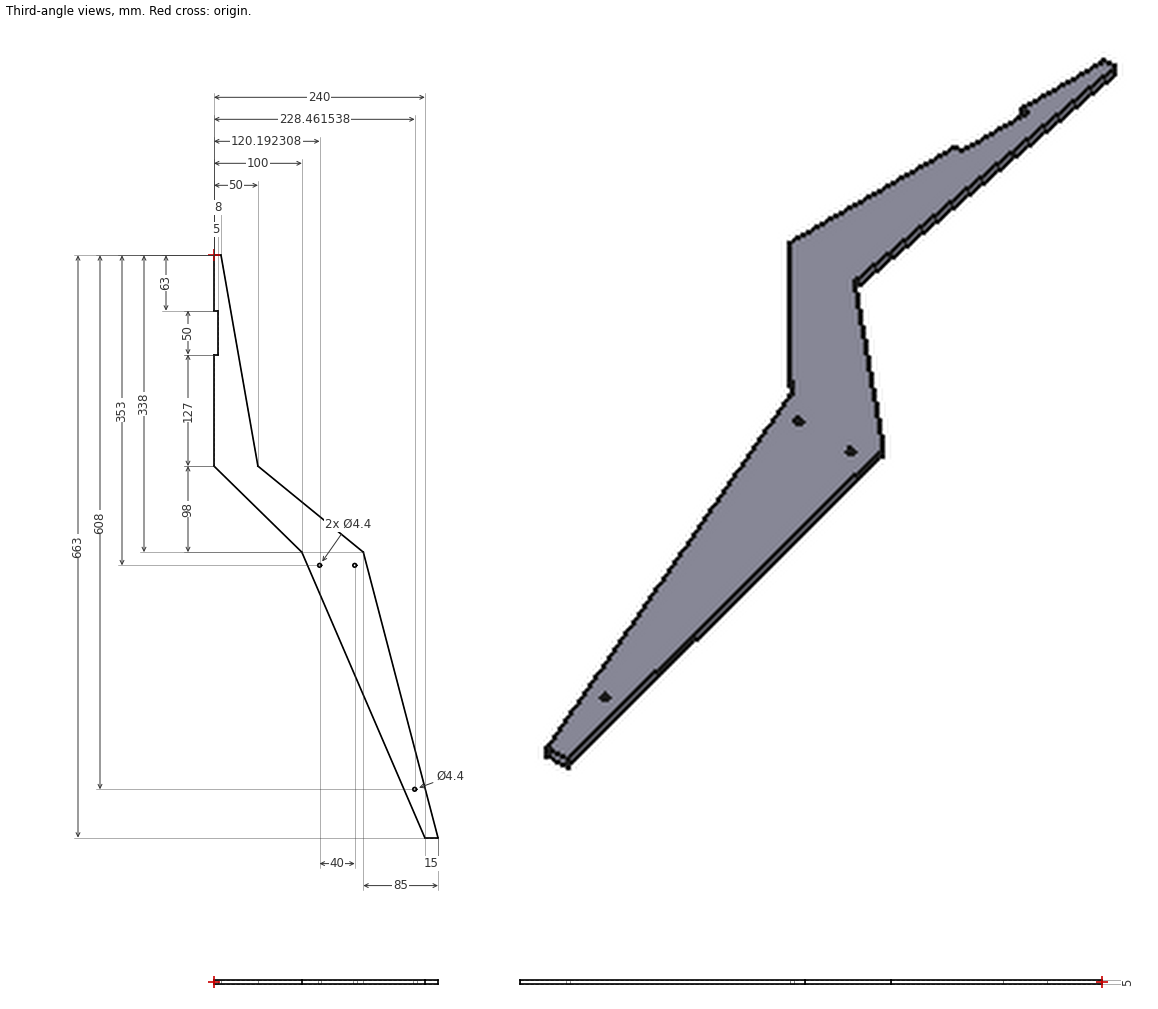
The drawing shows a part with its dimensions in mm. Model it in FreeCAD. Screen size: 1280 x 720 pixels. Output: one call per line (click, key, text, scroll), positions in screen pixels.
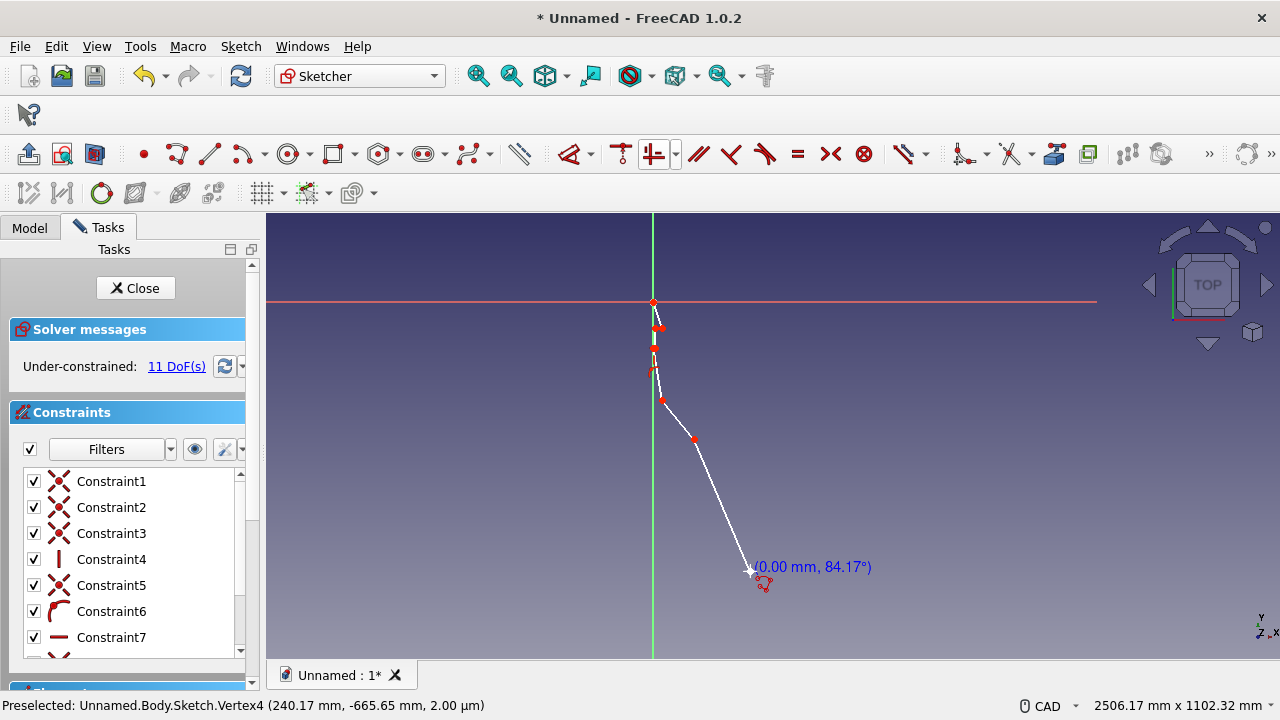
scroll(756, 571, up, 5)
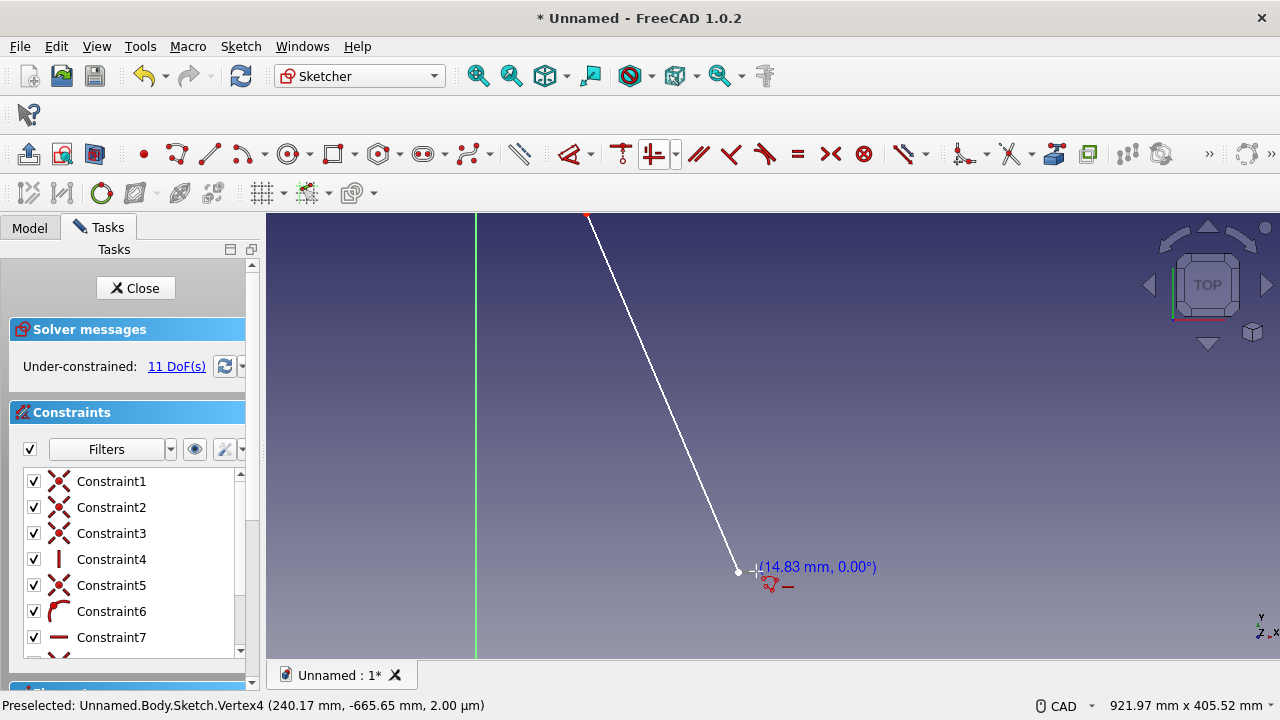
click(756, 570)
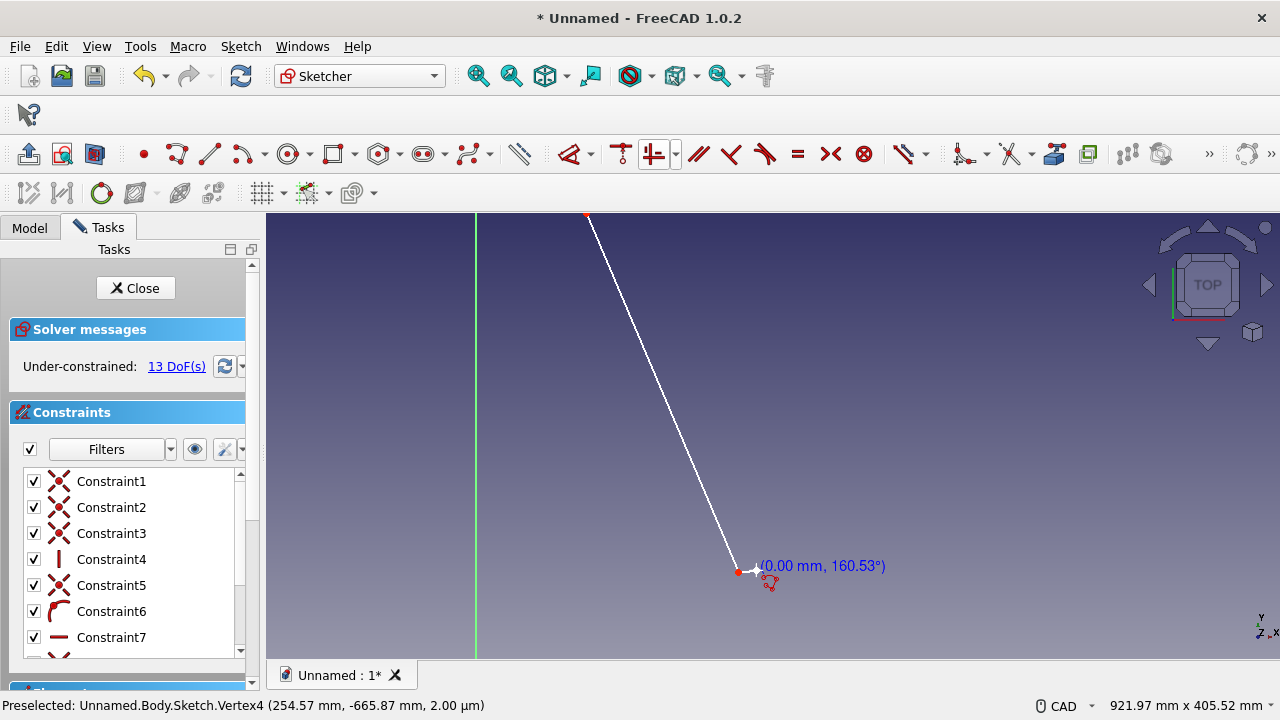
scroll(756, 571, down, 5)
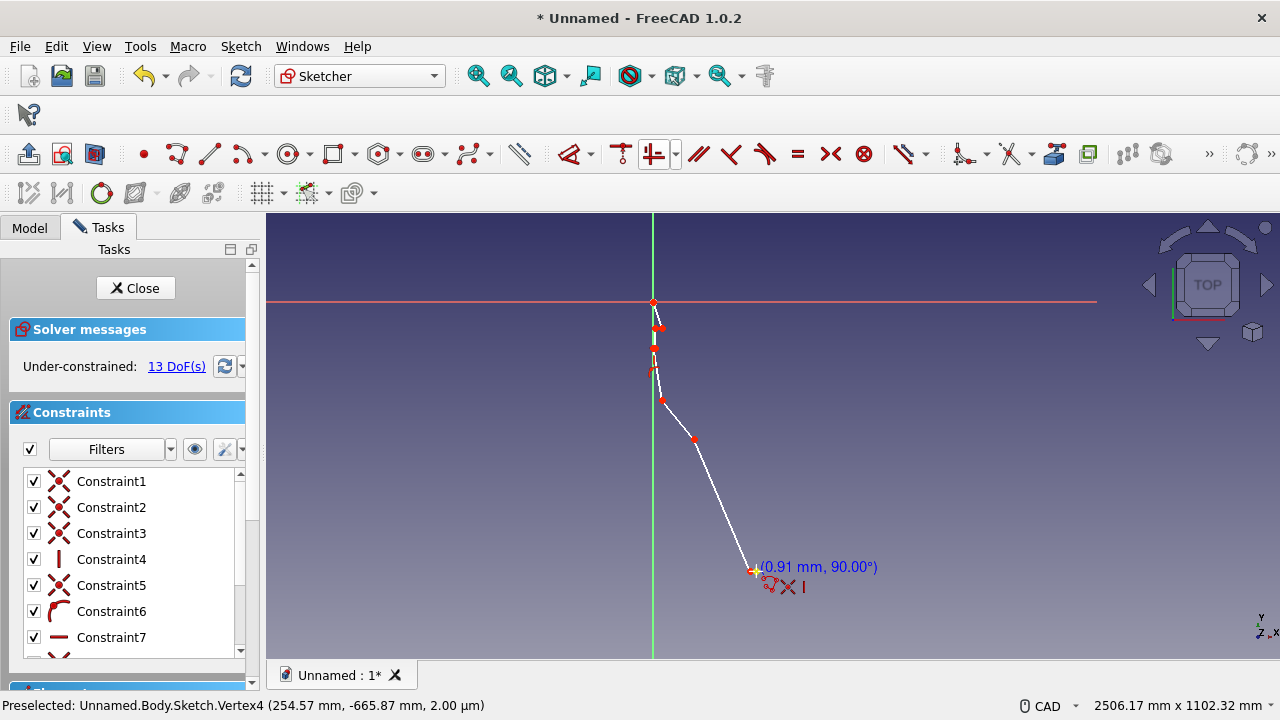
click(722, 439)
click(674, 400)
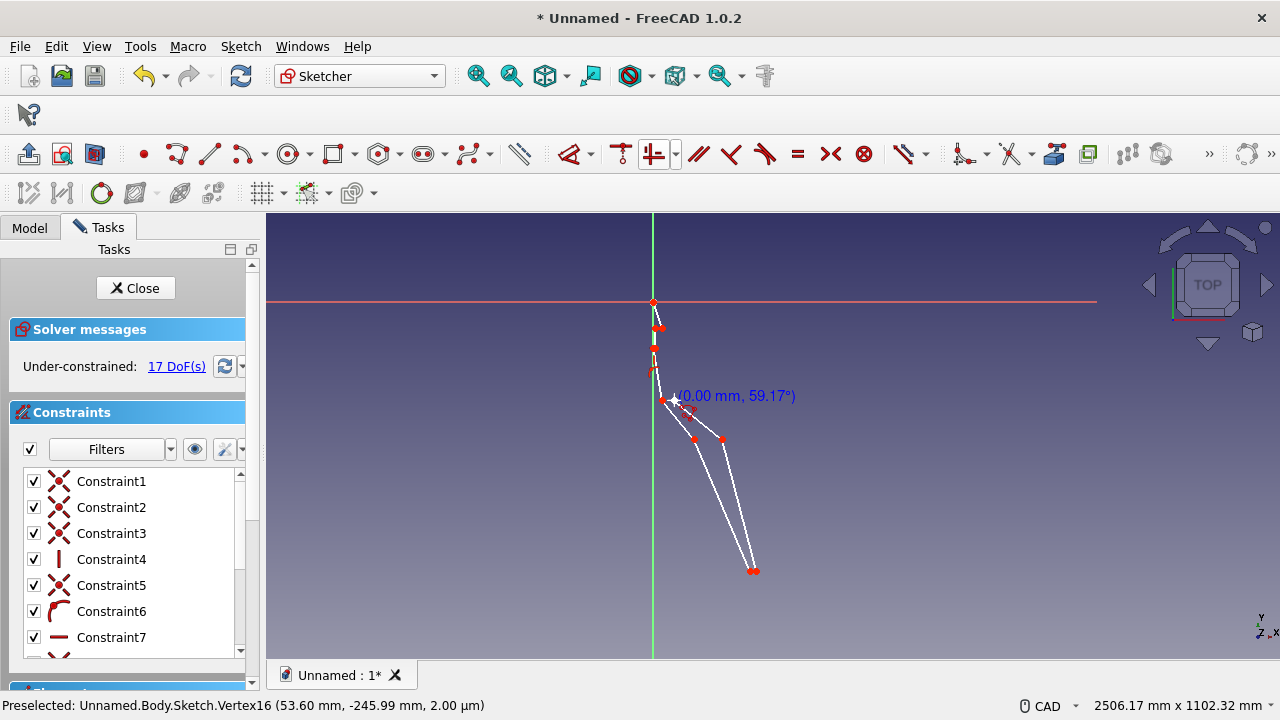
scroll(657, 302, up, 8)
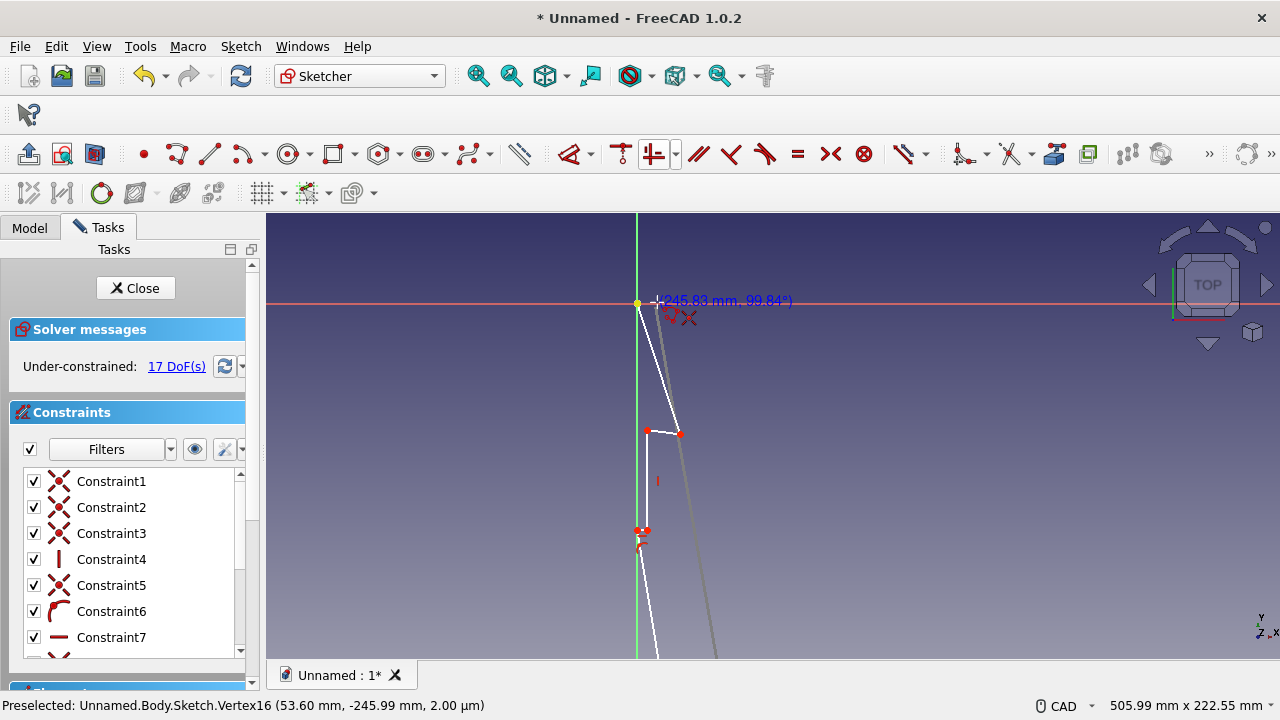
click(653, 313)
click(637, 304)
key(Escape)
key(Escape)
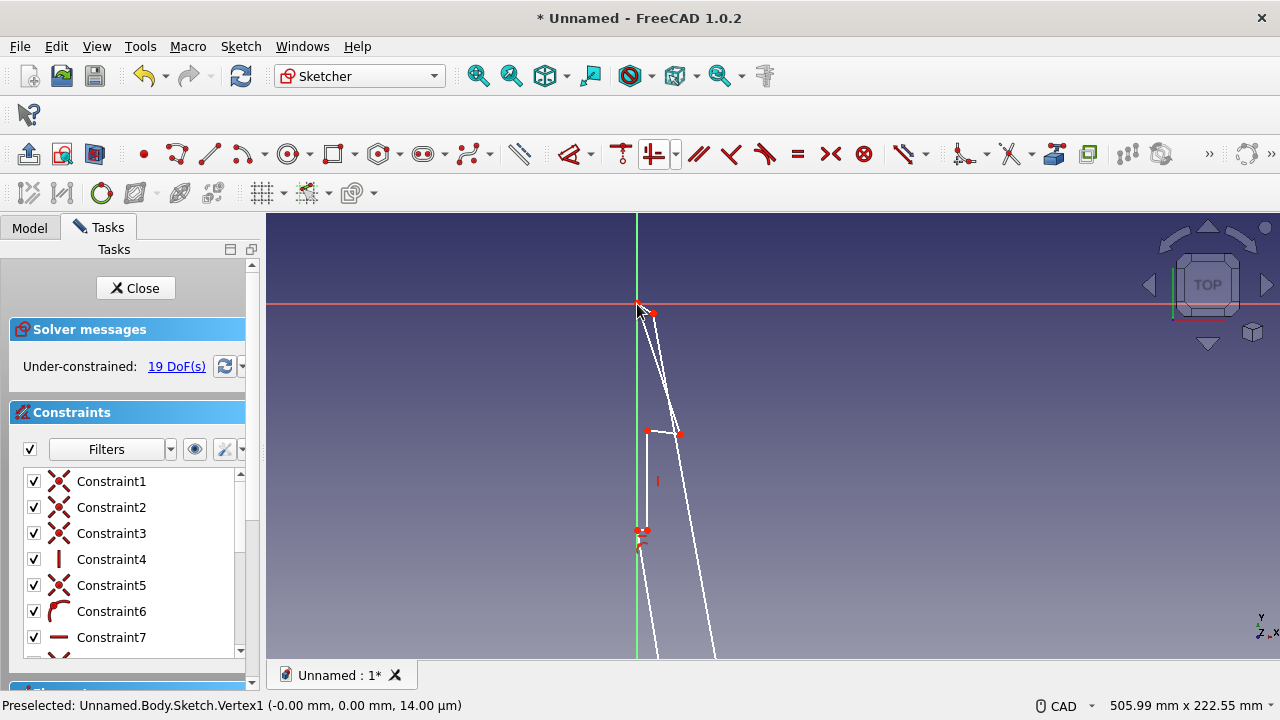
scroll(646, 330, up, 3)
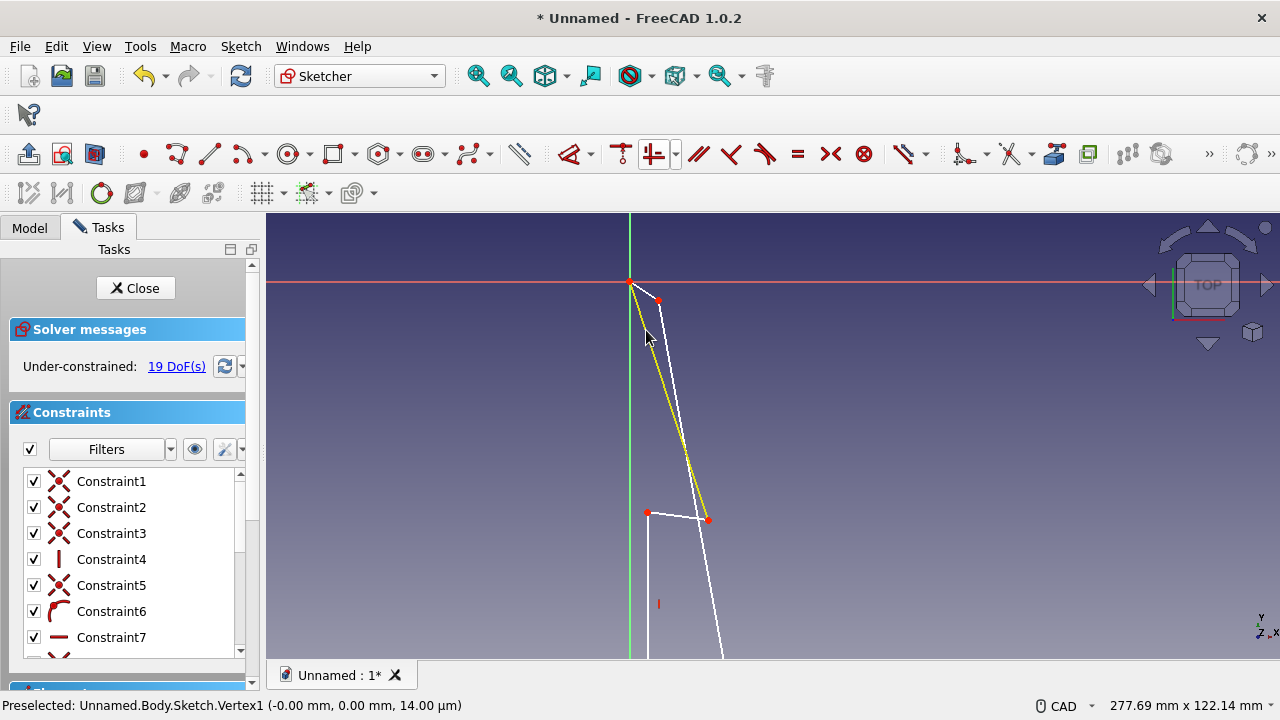
click(645, 329)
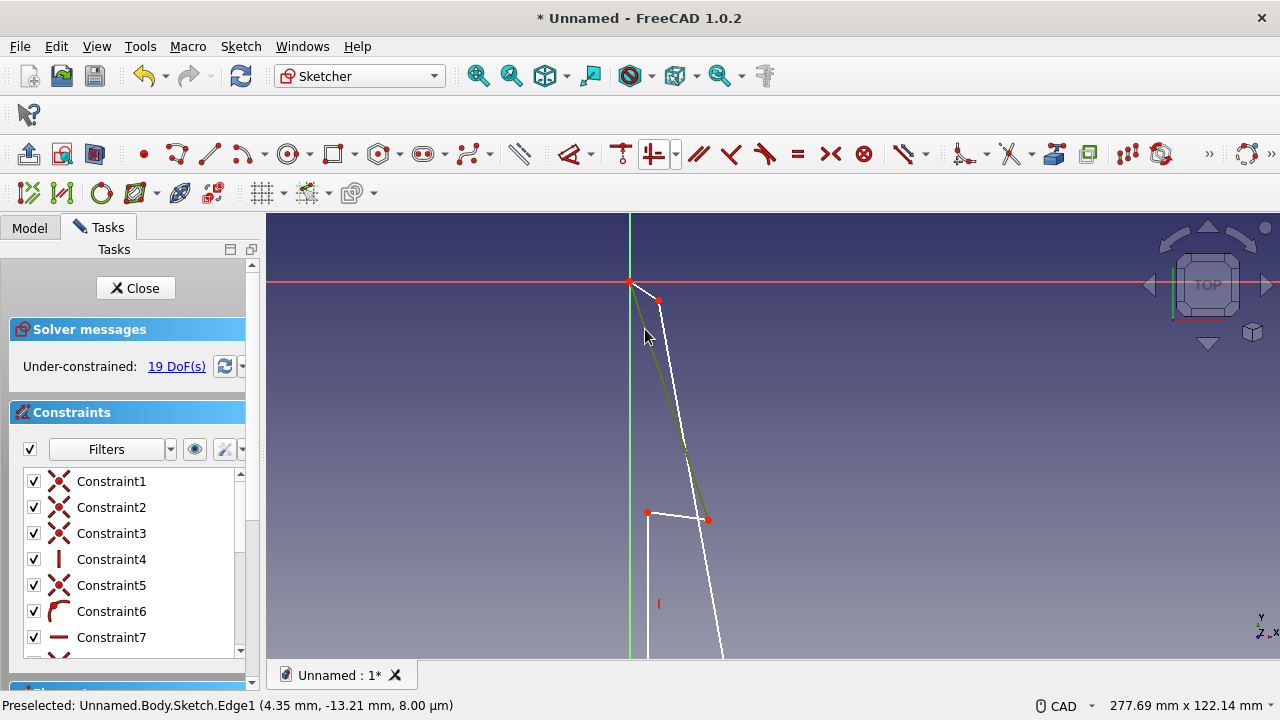
click(676, 154)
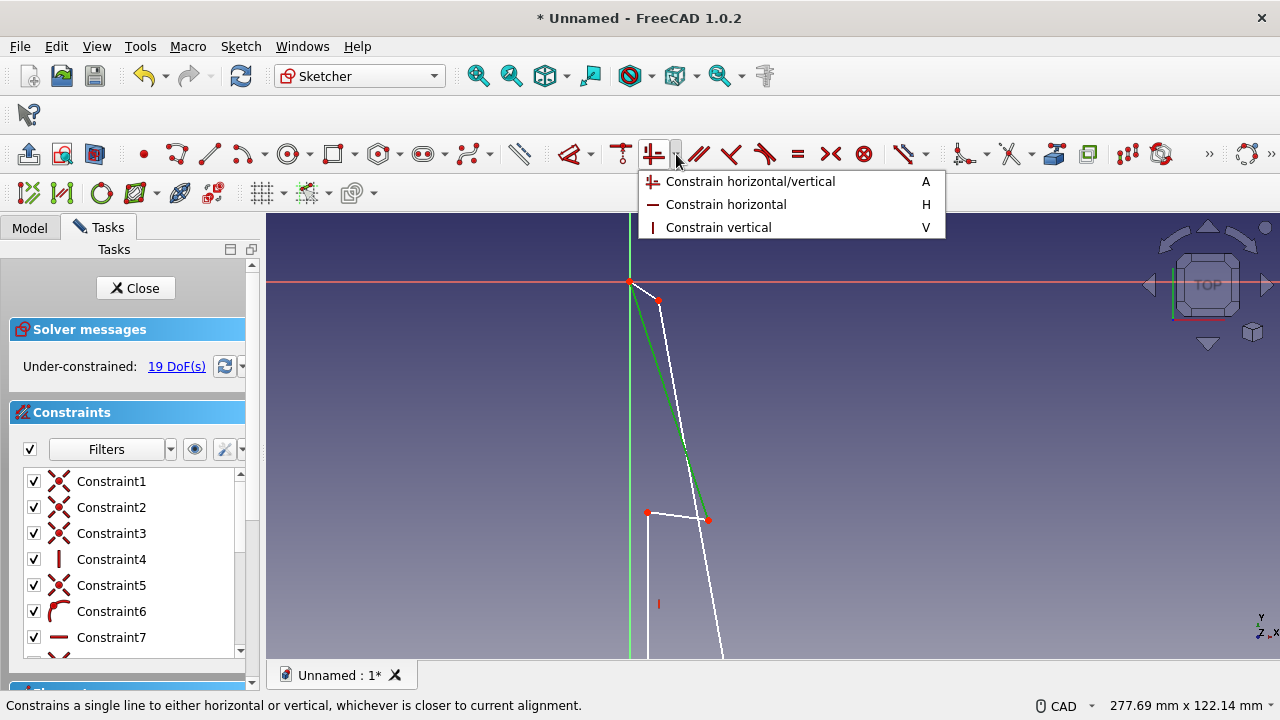
click(792, 228)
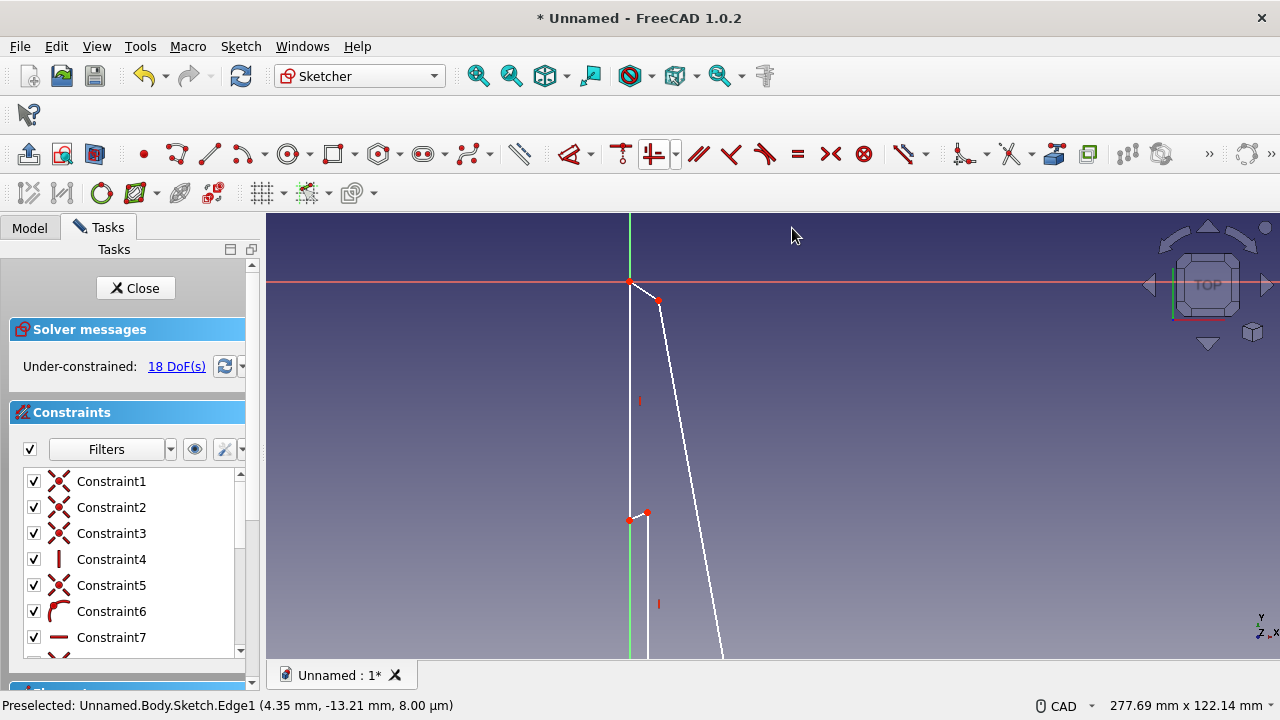
scroll(639, 516, up, 3)